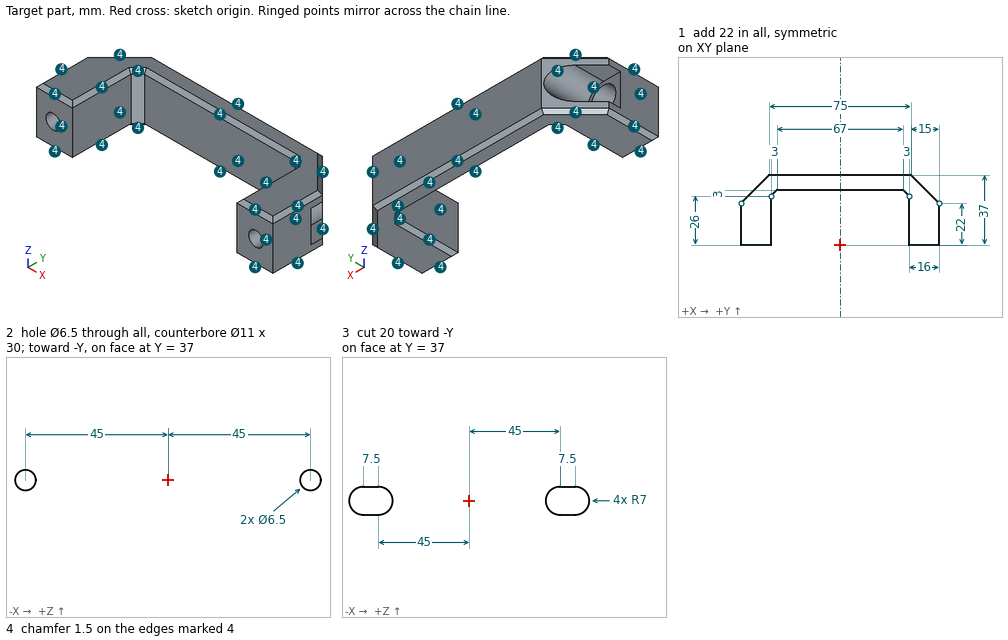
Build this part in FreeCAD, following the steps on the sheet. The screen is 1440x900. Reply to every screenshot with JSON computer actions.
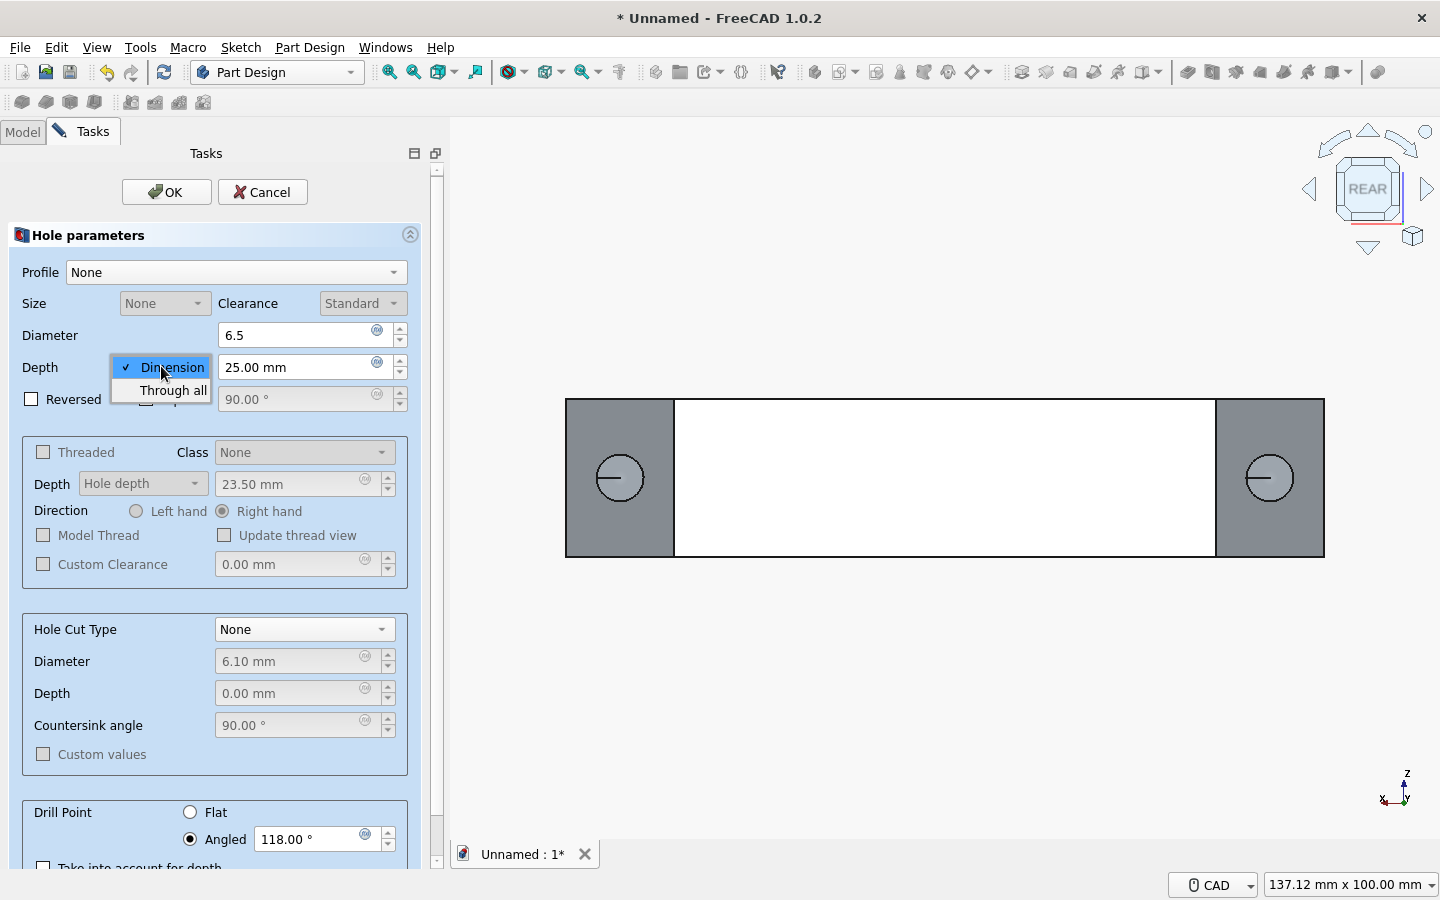
{"action": "left_click", "coordinate": [160, 390]}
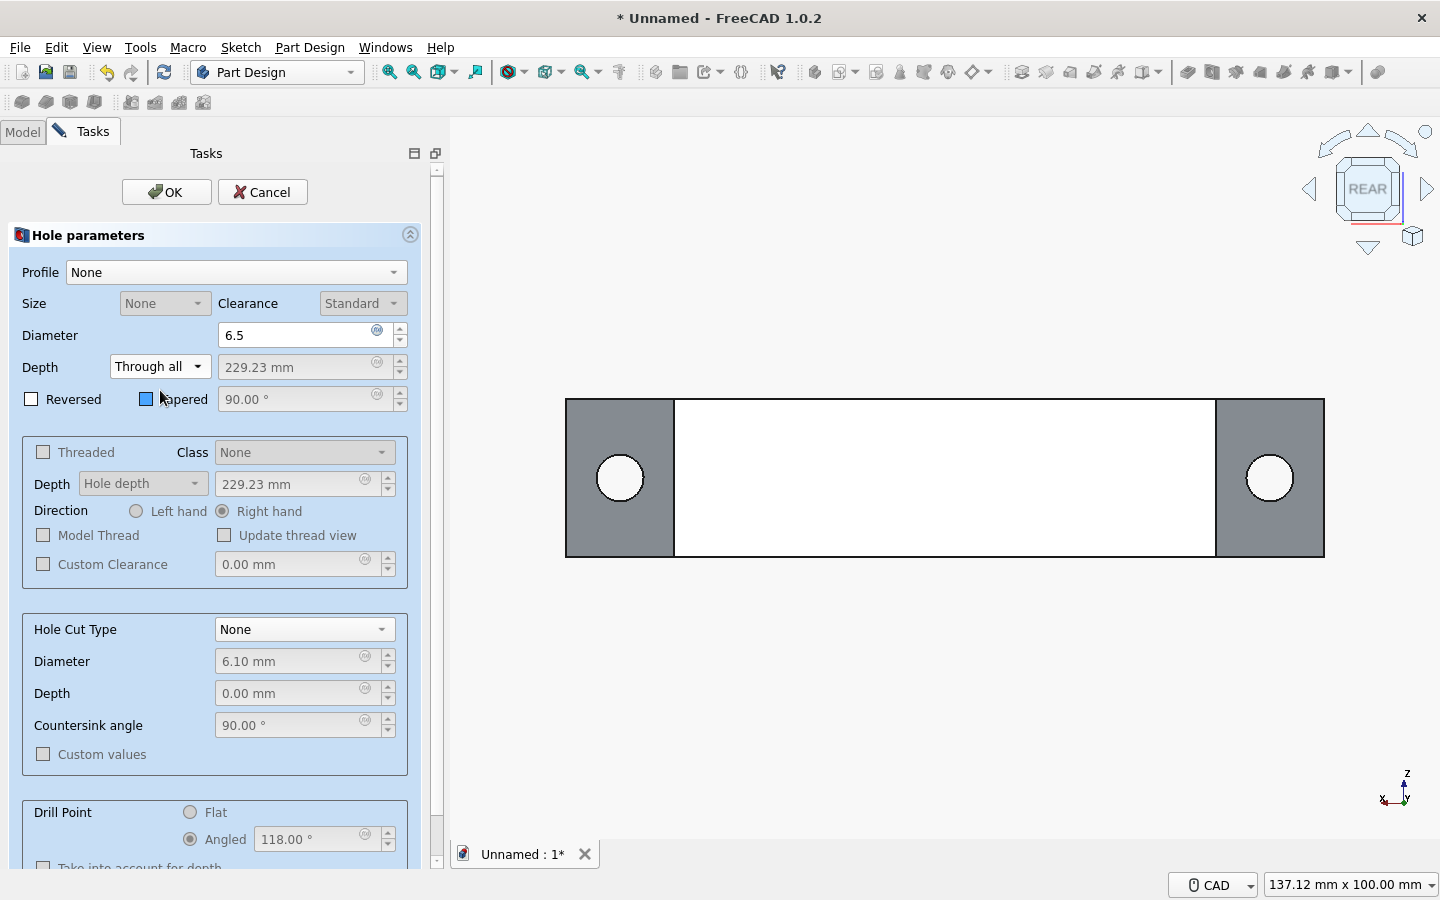
{"action": "left_click", "coordinate": [306, 630]}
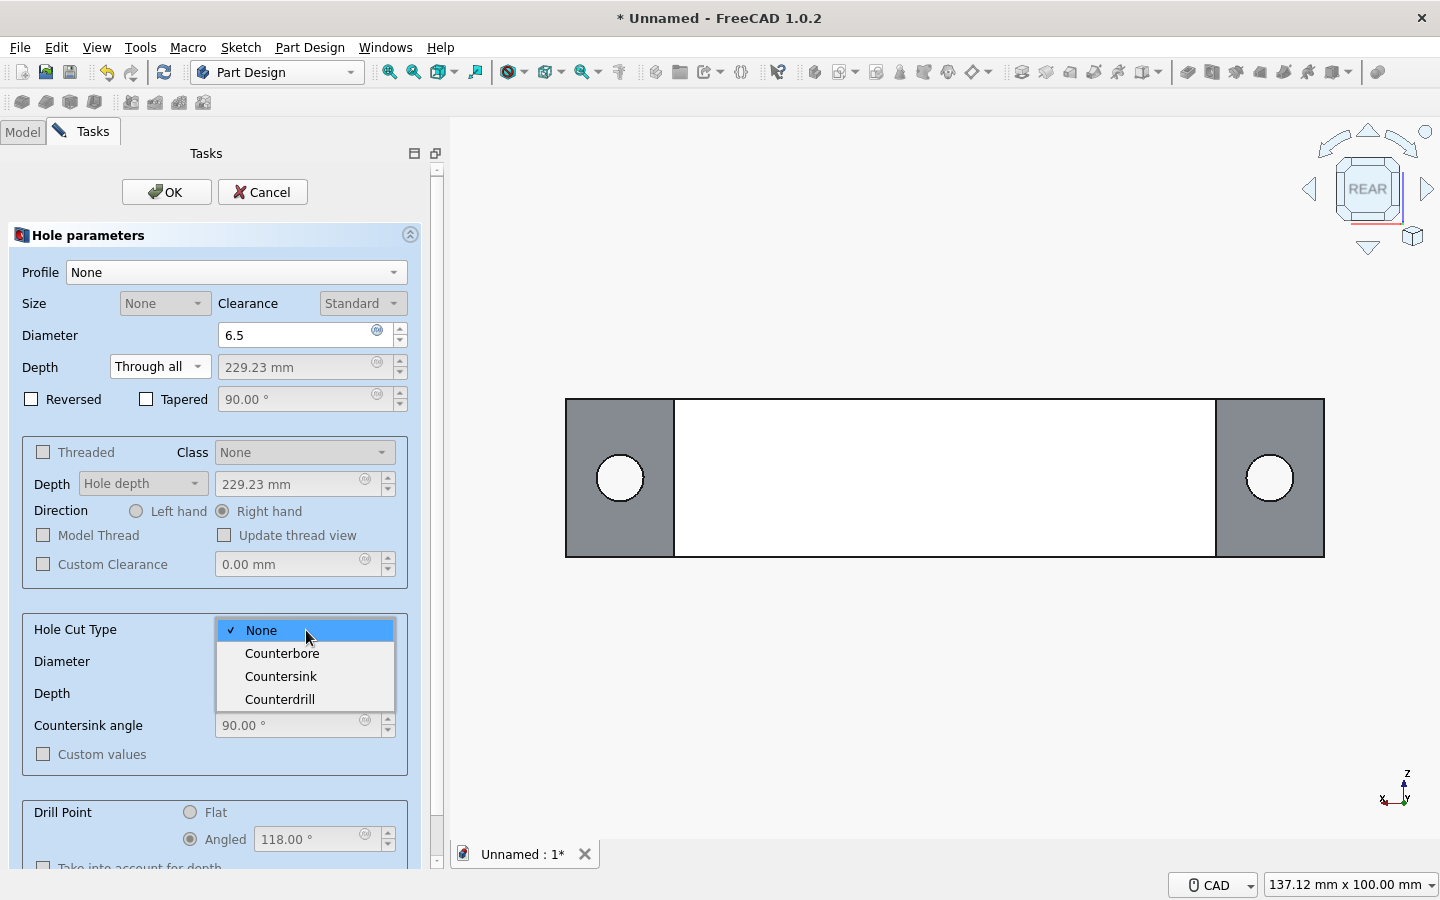
{"action": "left_click", "coordinate": [304, 654]}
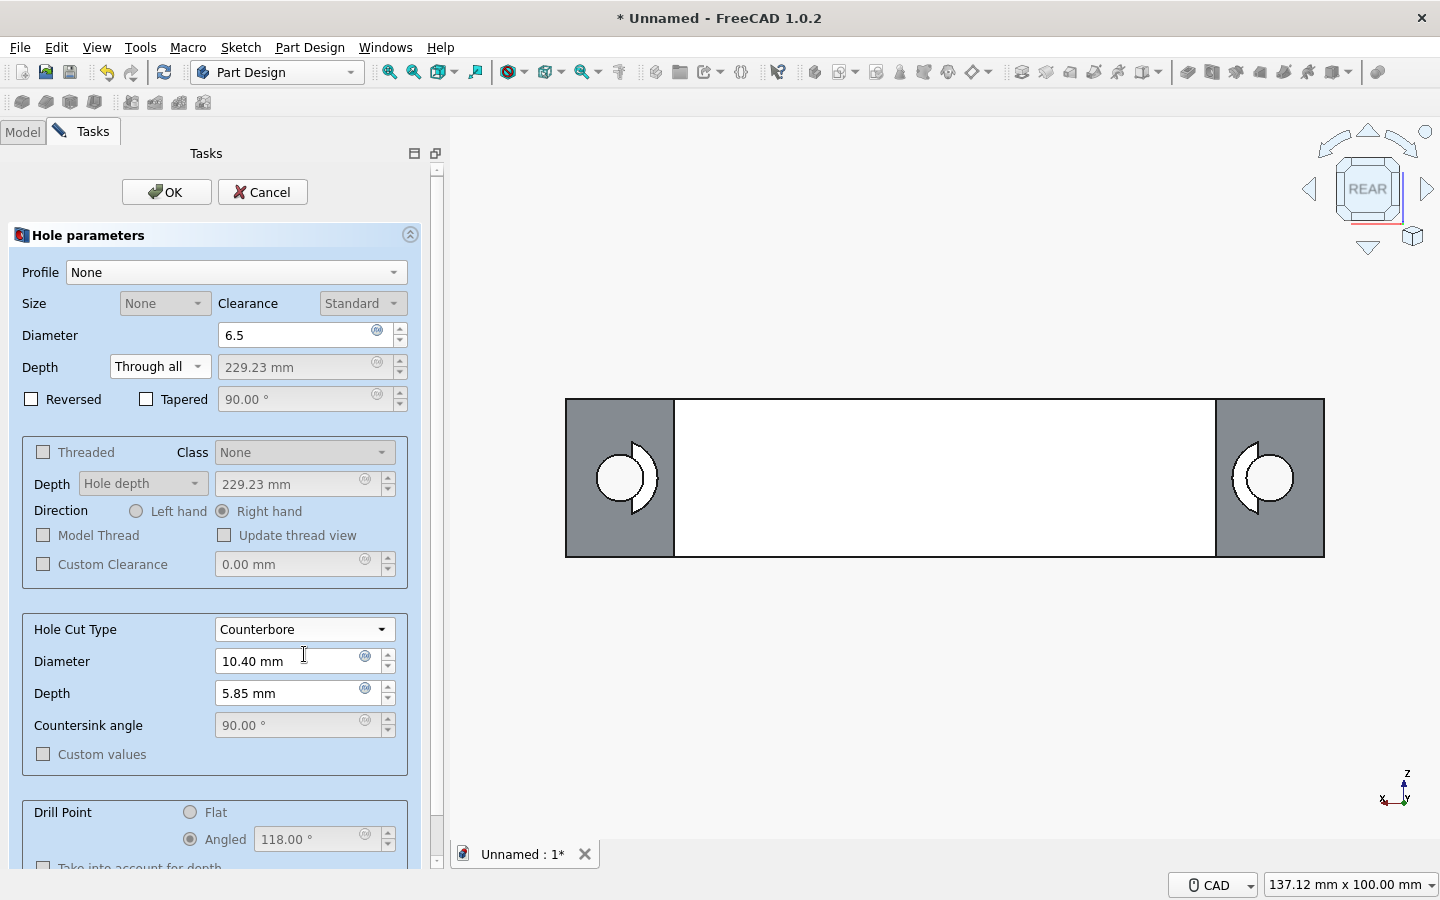
{"action": "triple_click", "coordinate": [298, 661]}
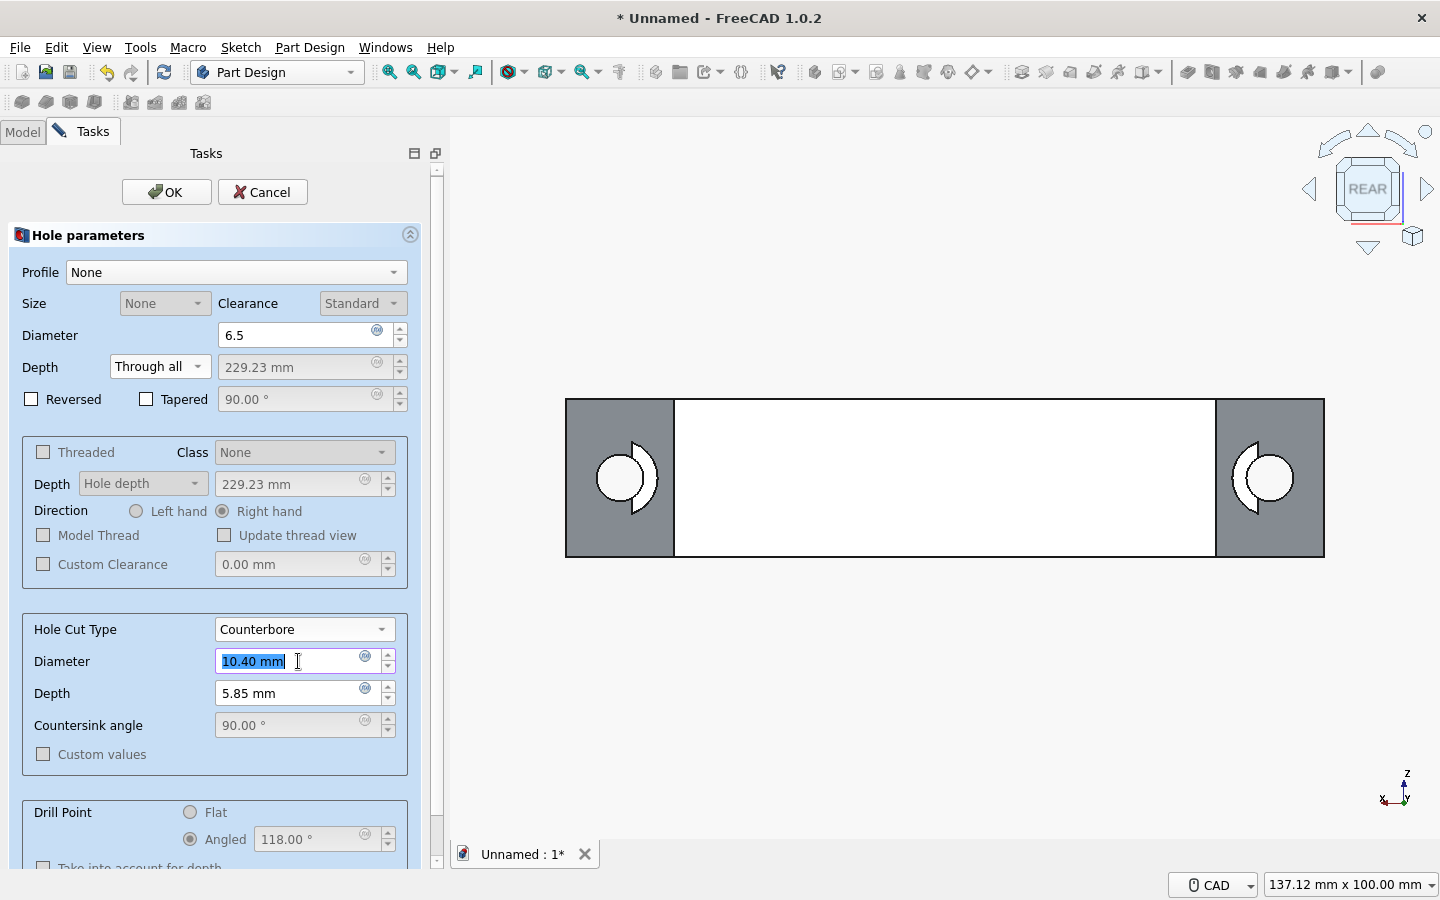
{"action": "type", "text": "11"}
{"action": "key", "text": "Tab"}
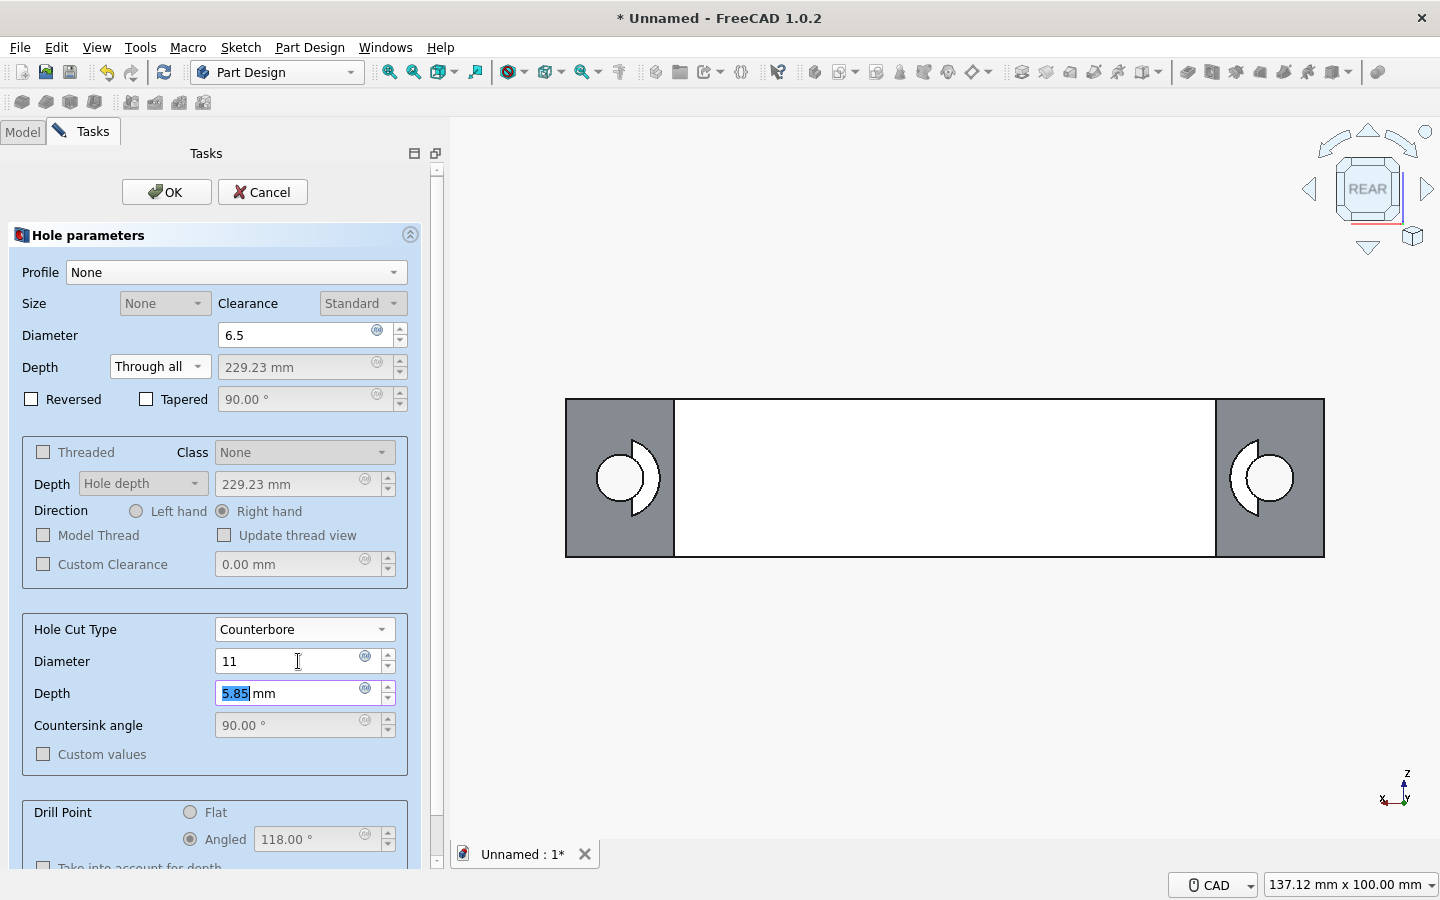
{"action": "type", "text": "30"}
{"action": "key", "text": "Tab"}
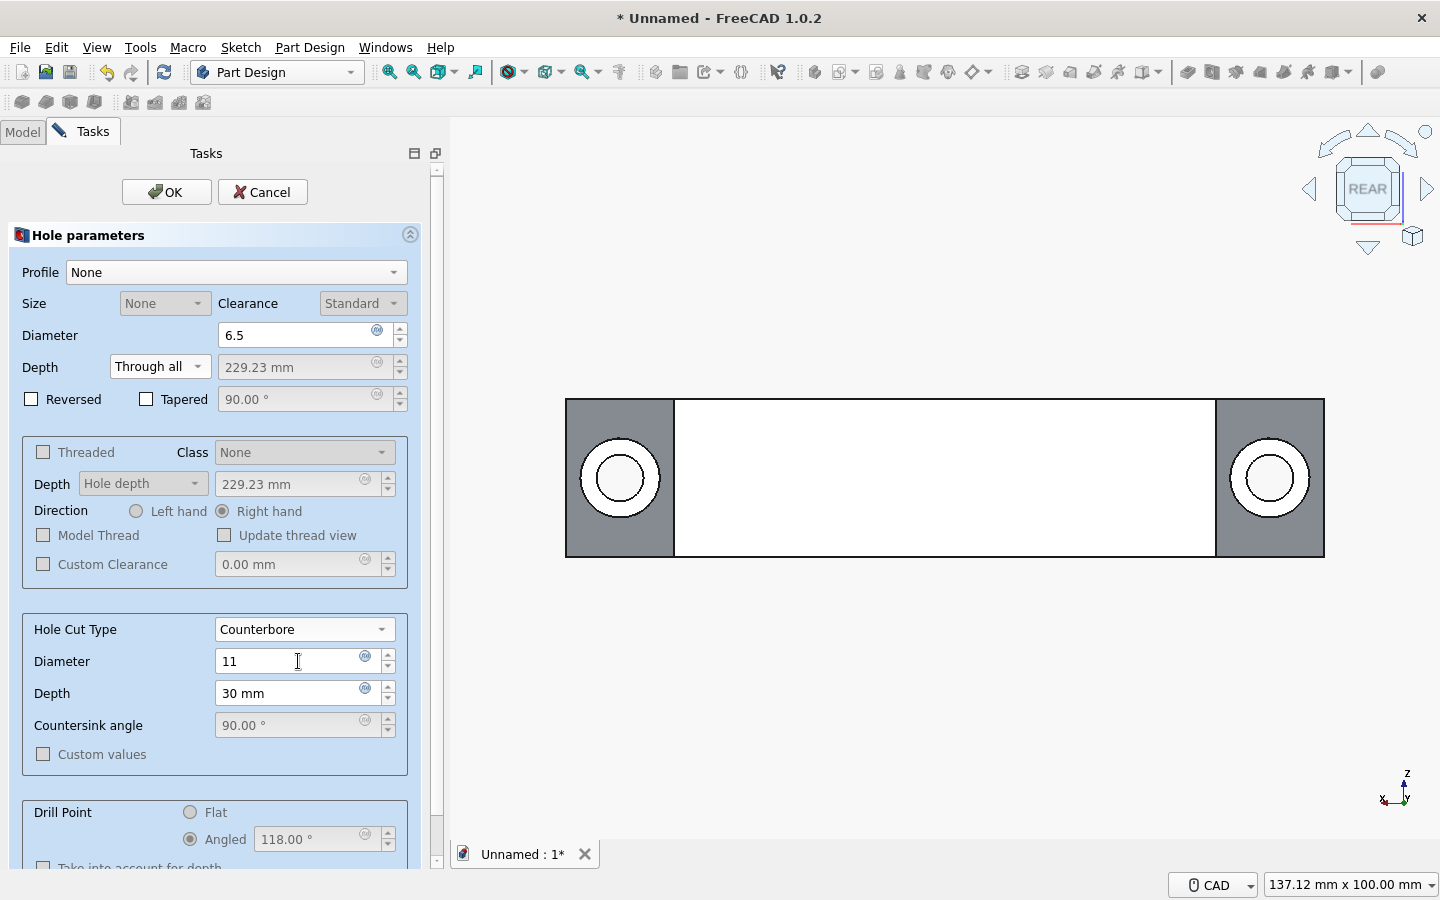
{"action": "left_click", "coordinate": [167, 192]}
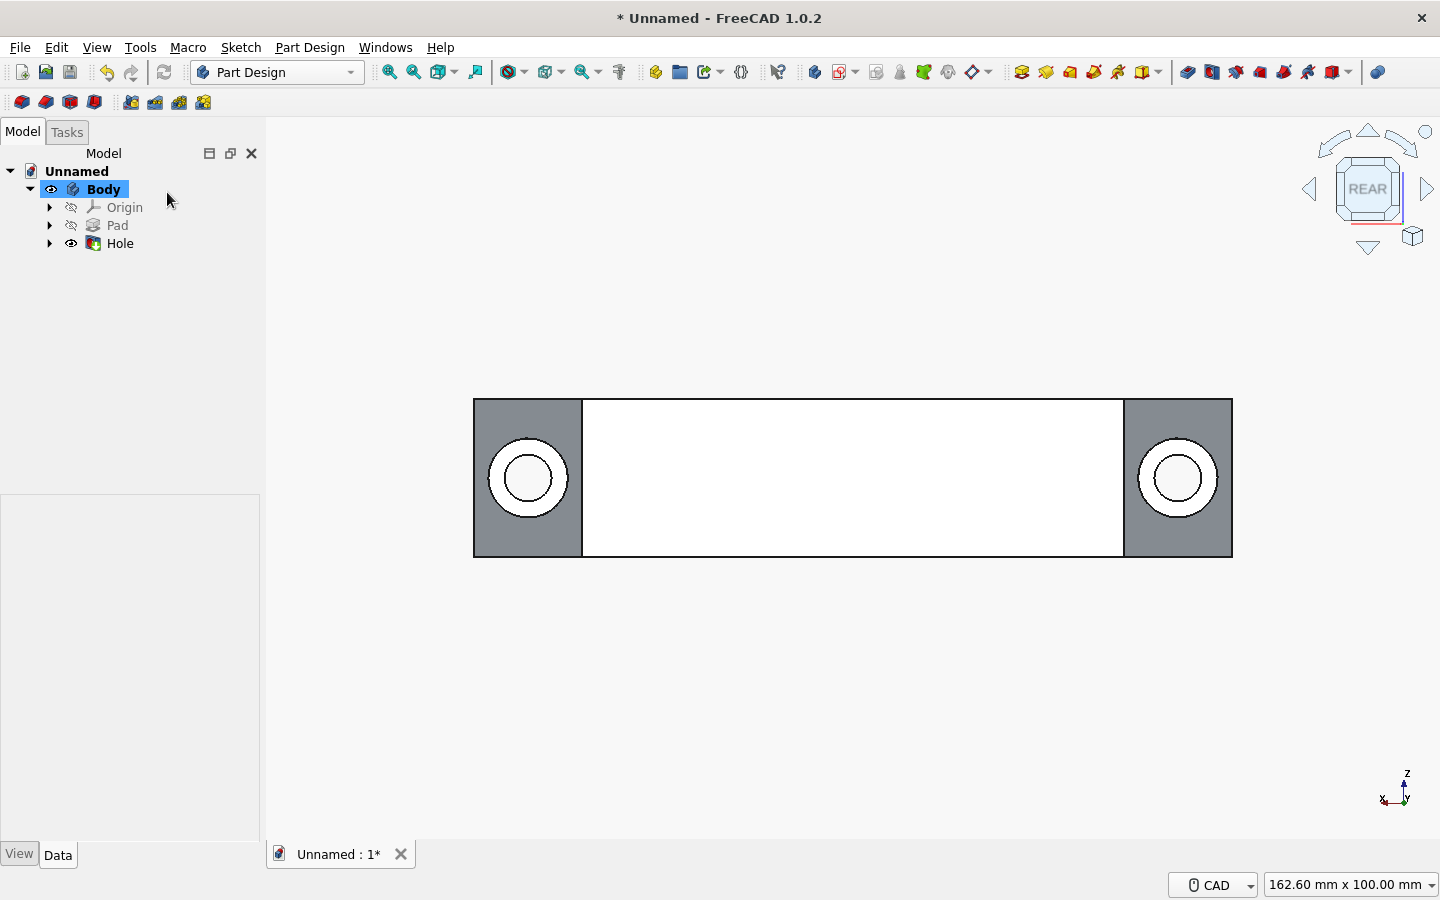
{"action": "left_click", "coordinate": [698, 477]}